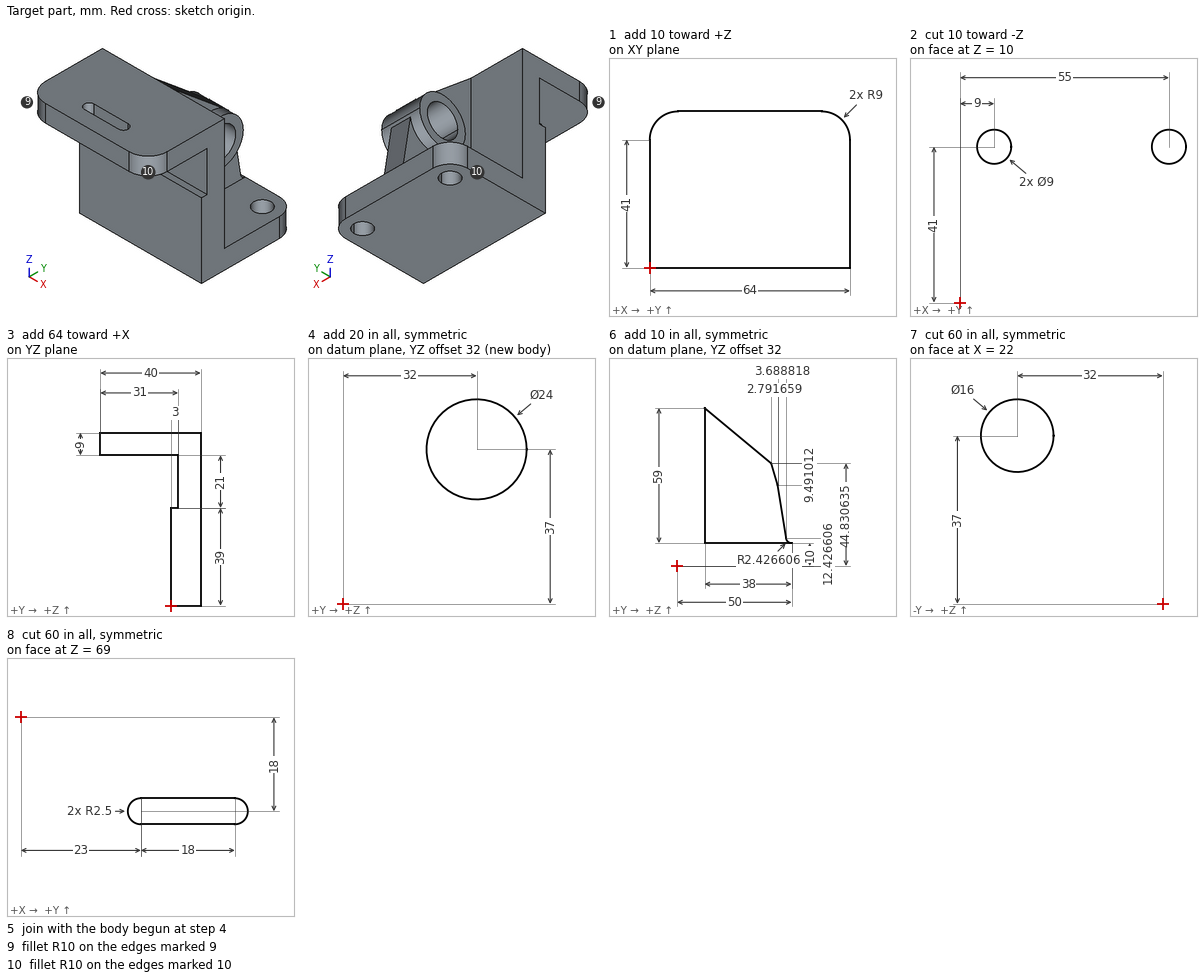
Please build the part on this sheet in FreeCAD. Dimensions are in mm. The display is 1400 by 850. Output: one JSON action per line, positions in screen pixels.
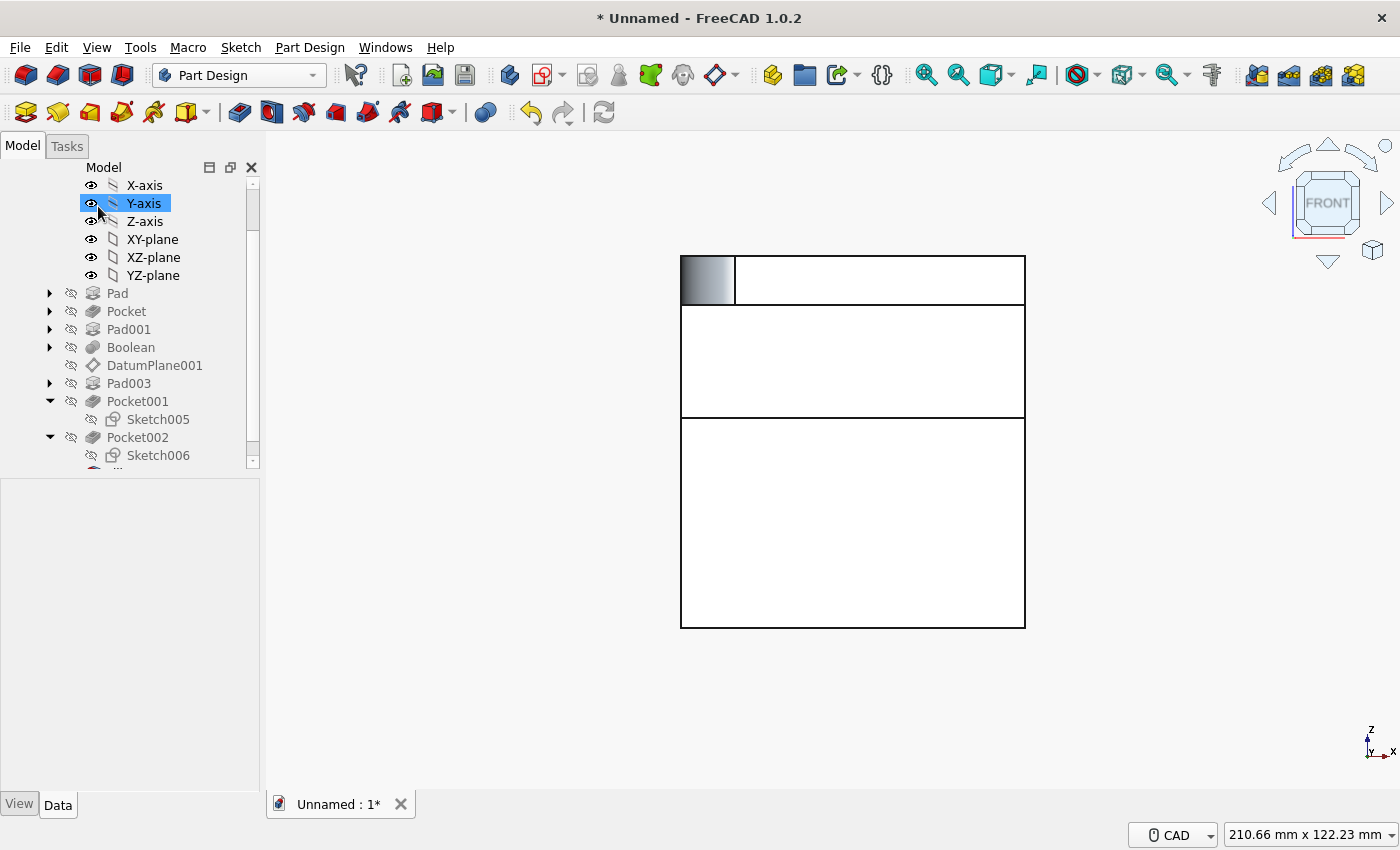
{"action": "left_click", "coordinate": [1025, 280]}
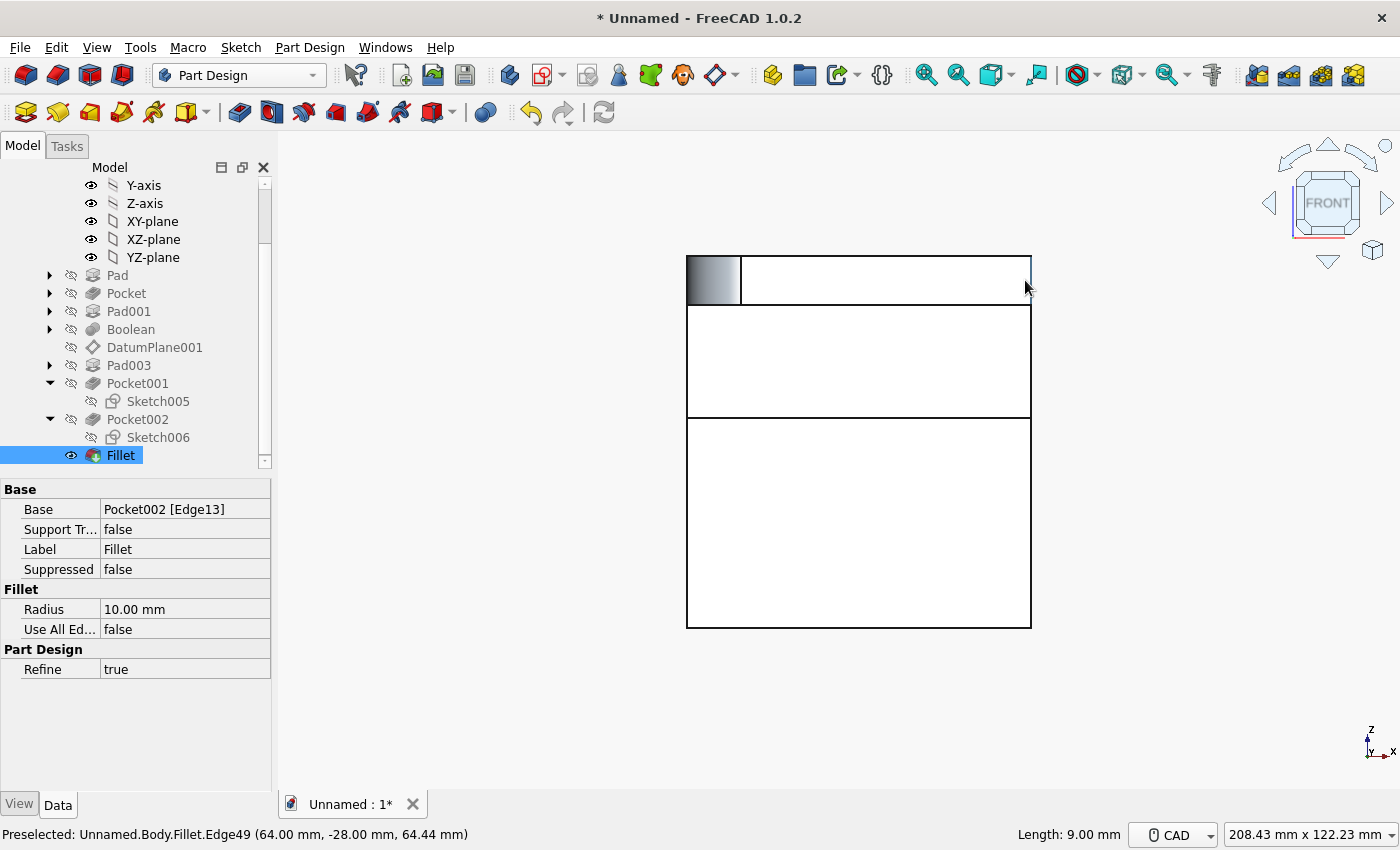
{"action": "left_click", "coordinate": [26, 76]}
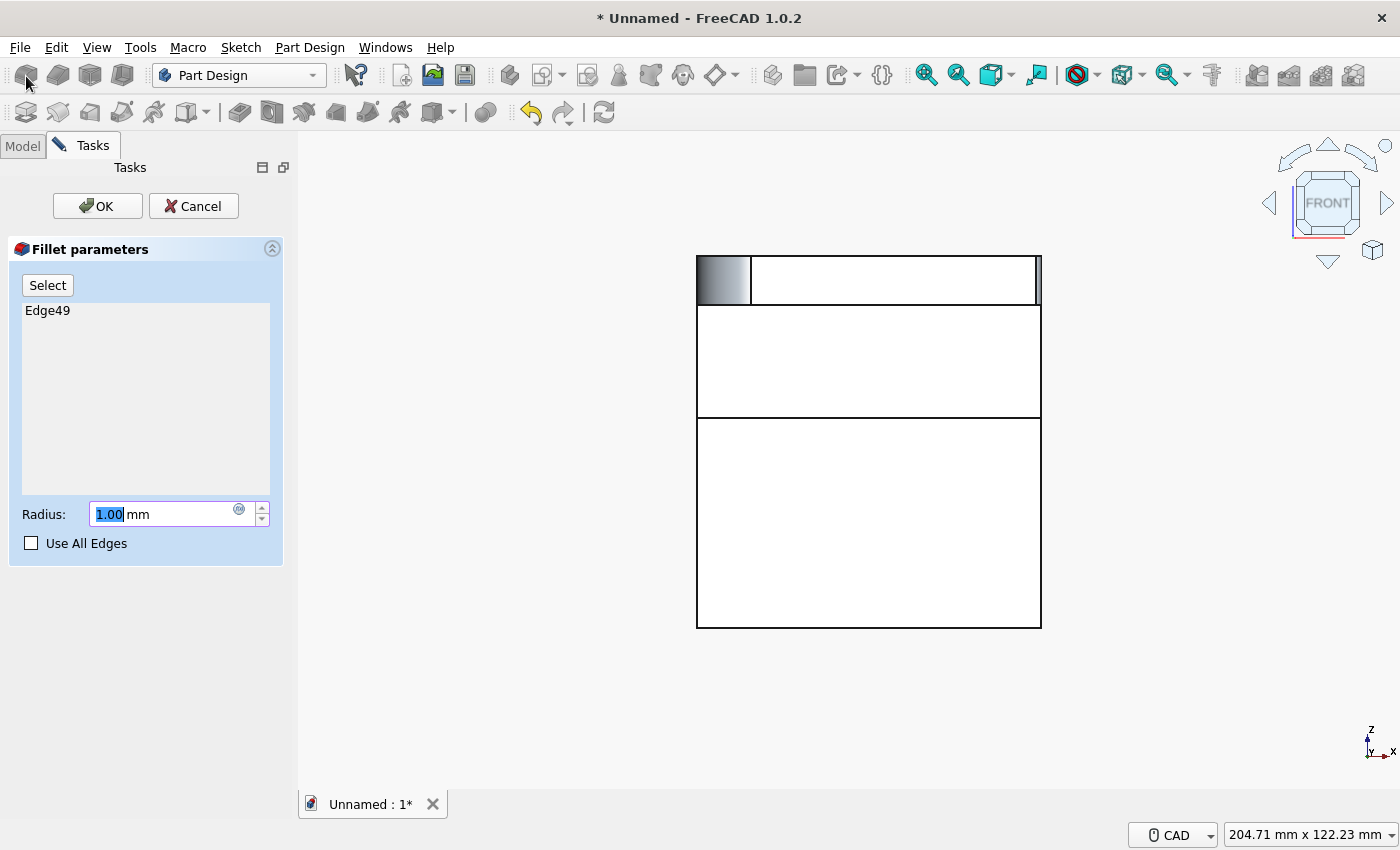
{"action": "type", "text": "10"}
{"action": "key", "text": "Tab"}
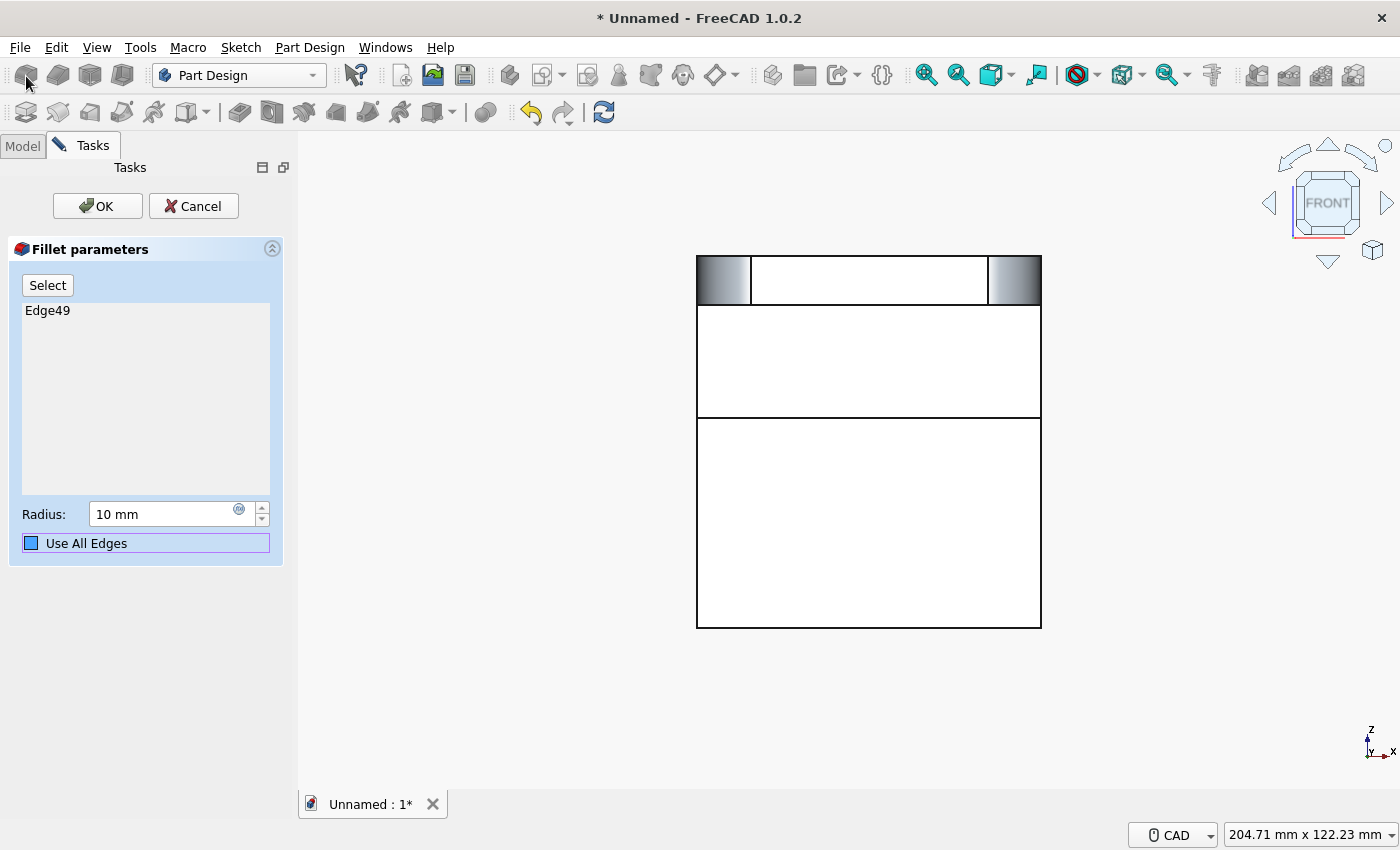
{"action": "left_click", "coordinate": [98, 206]}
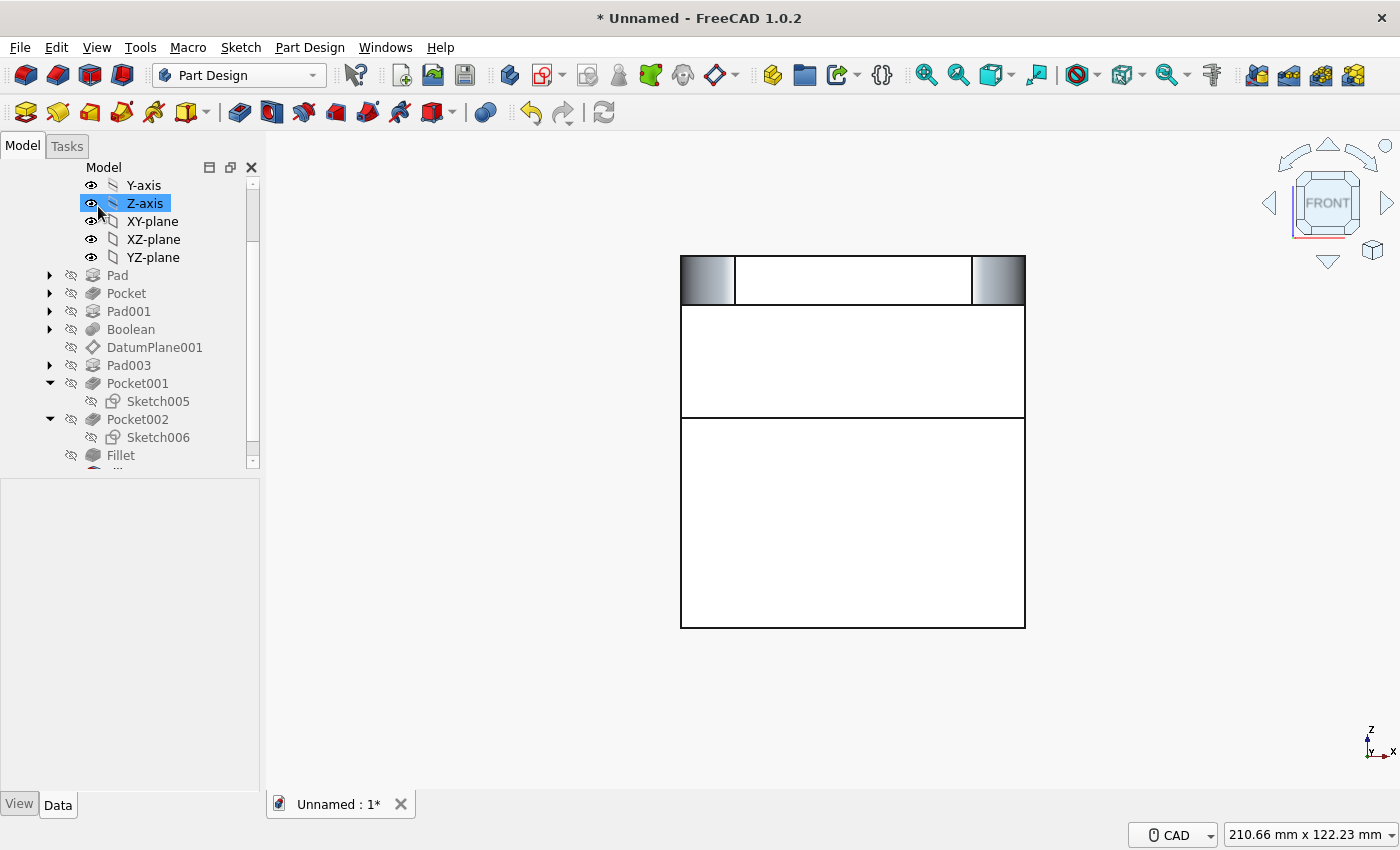
{"action": "key", "text": "0"}